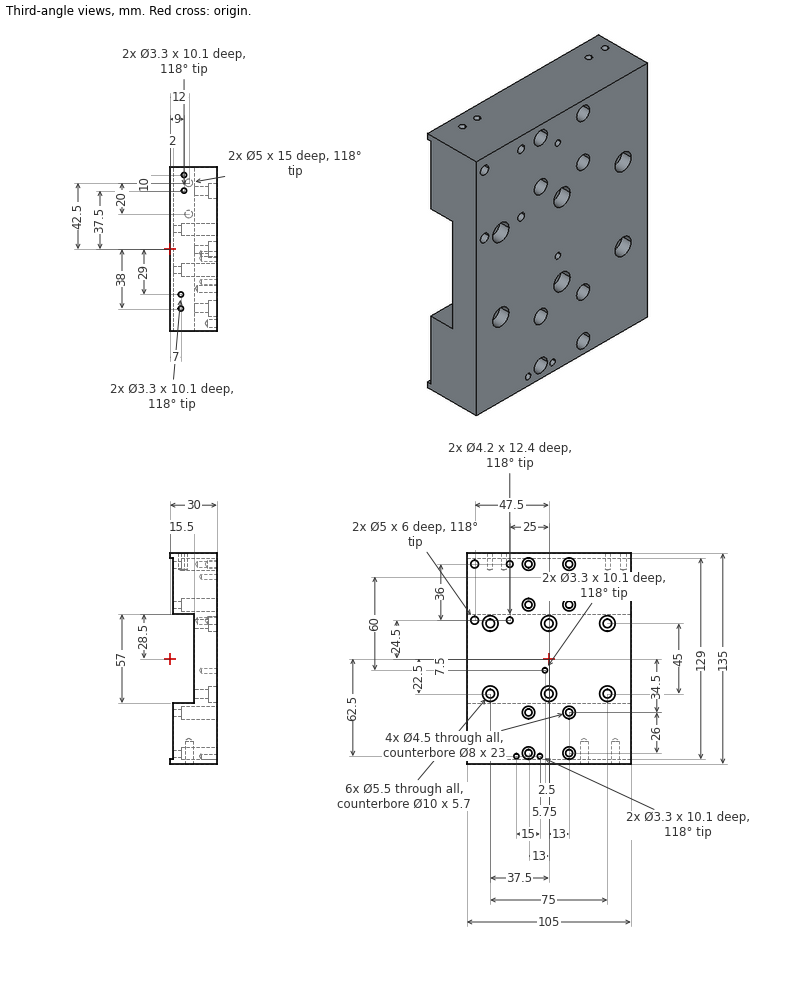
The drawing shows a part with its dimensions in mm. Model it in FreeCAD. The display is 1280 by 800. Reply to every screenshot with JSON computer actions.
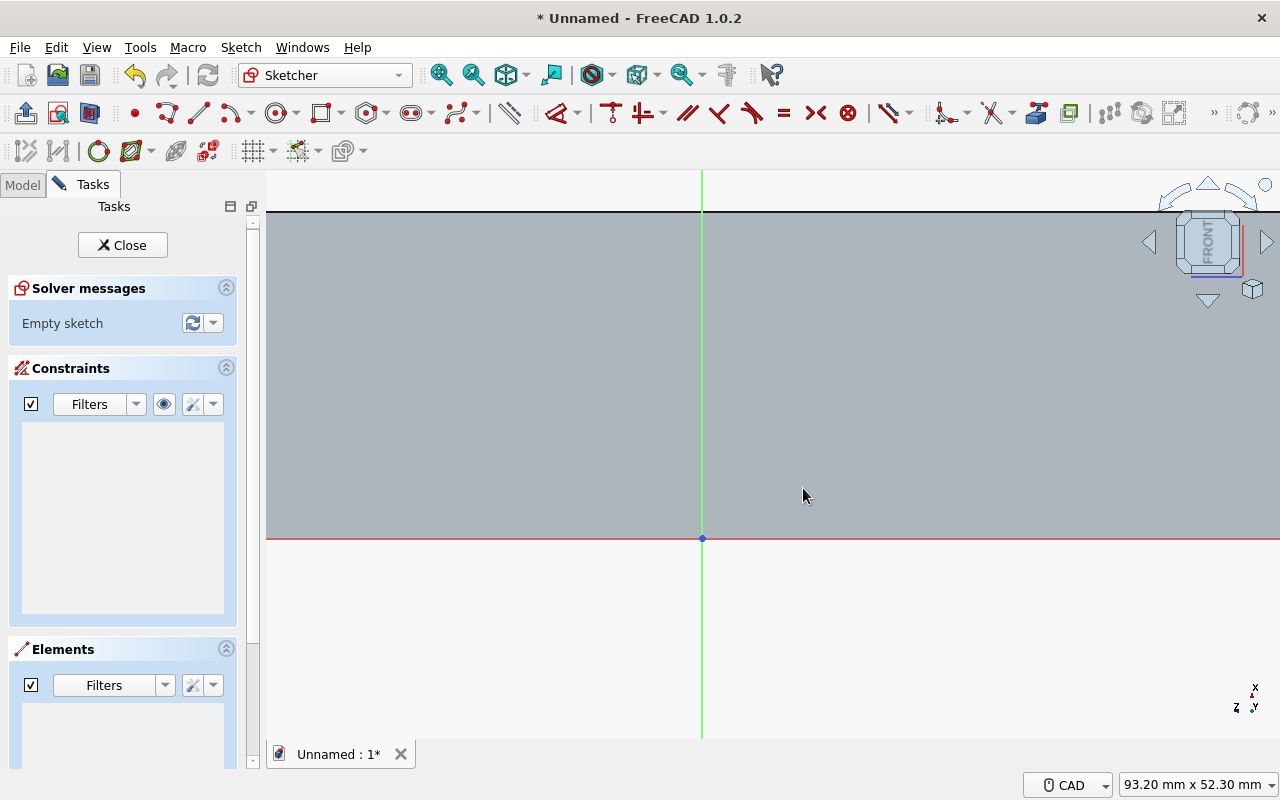
{"action": "left_click", "coordinate": [322, 114]}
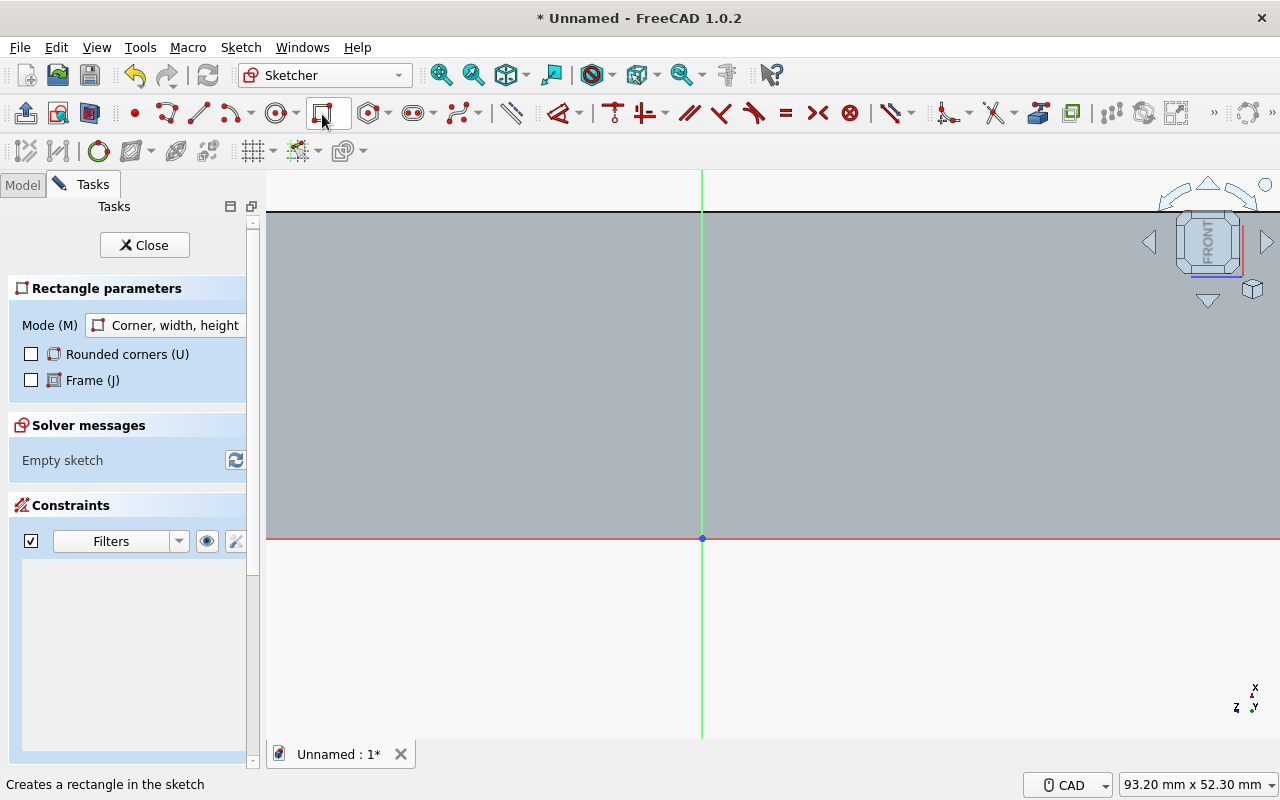
{"action": "left_click", "coordinate": [392, 370]}
{"action": "left_click", "coordinate": [1012, 539]}
{"action": "key", "text": "Escape"}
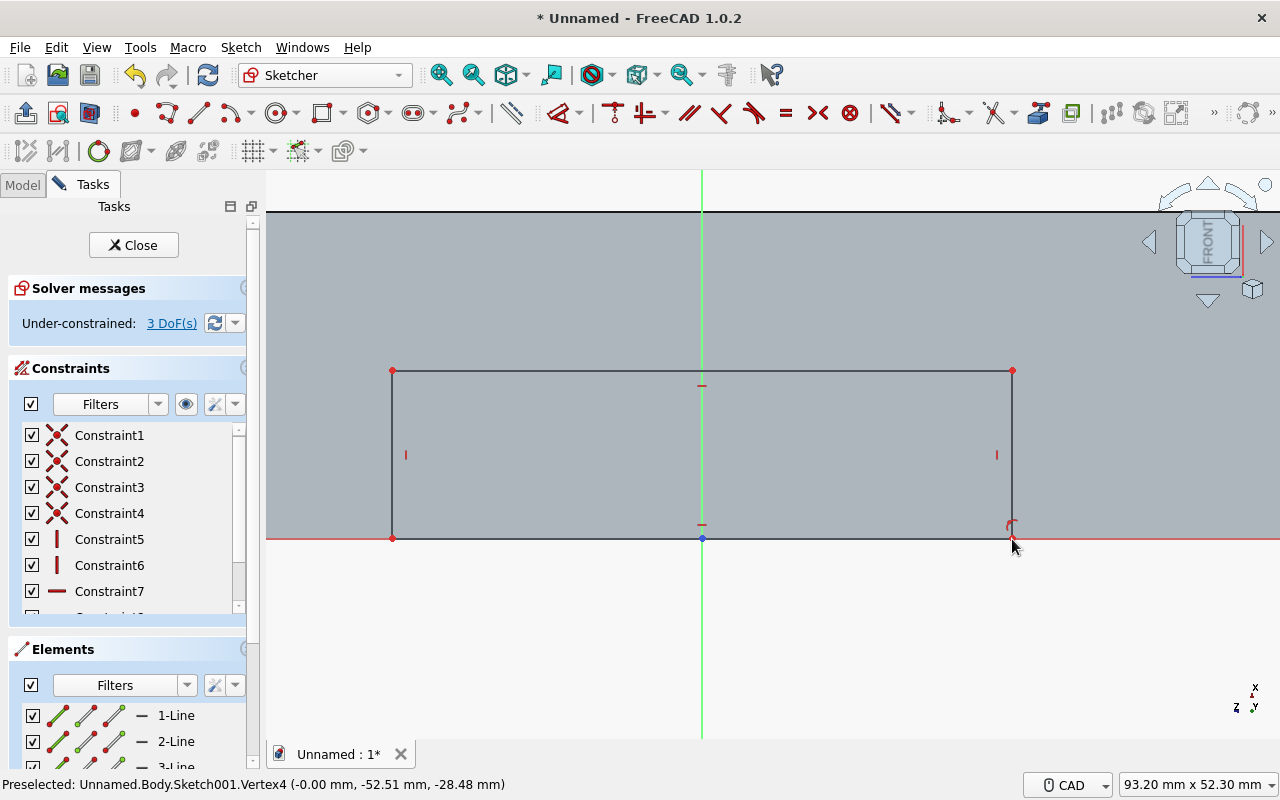
{"action": "left_click", "coordinate": [558, 114]}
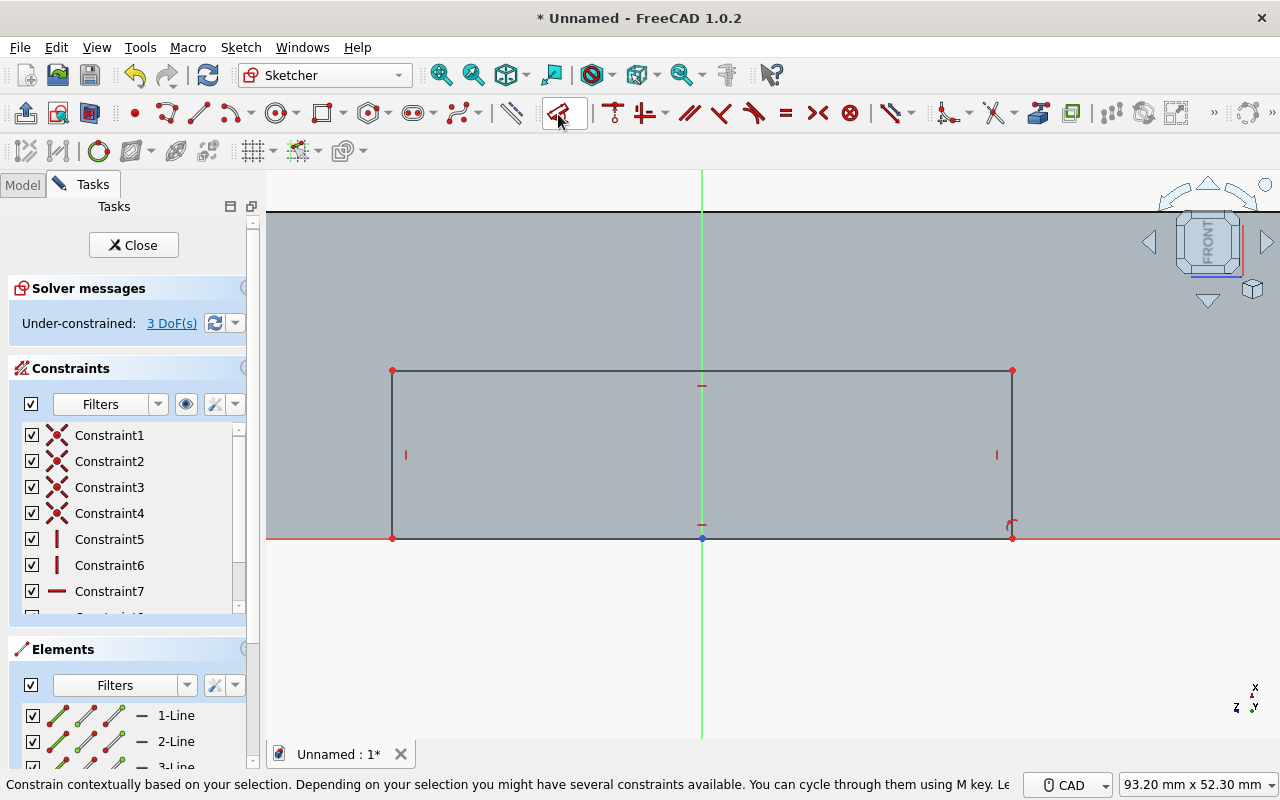
{"action": "left_click", "coordinate": [578, 539]}
{"action": "left_click", "coordinate": [559, 573]}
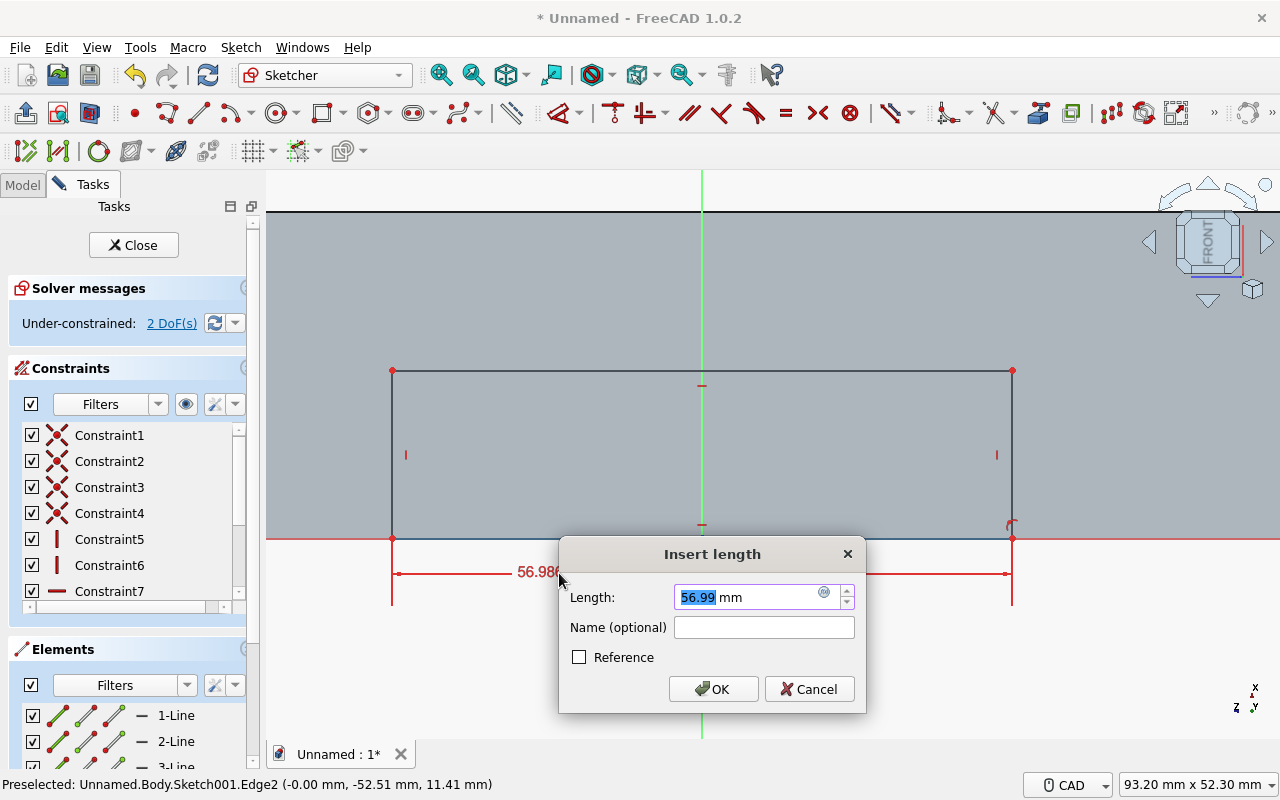
{"action": "type", "text": "57"}
{"action": "key", "text": "Return"}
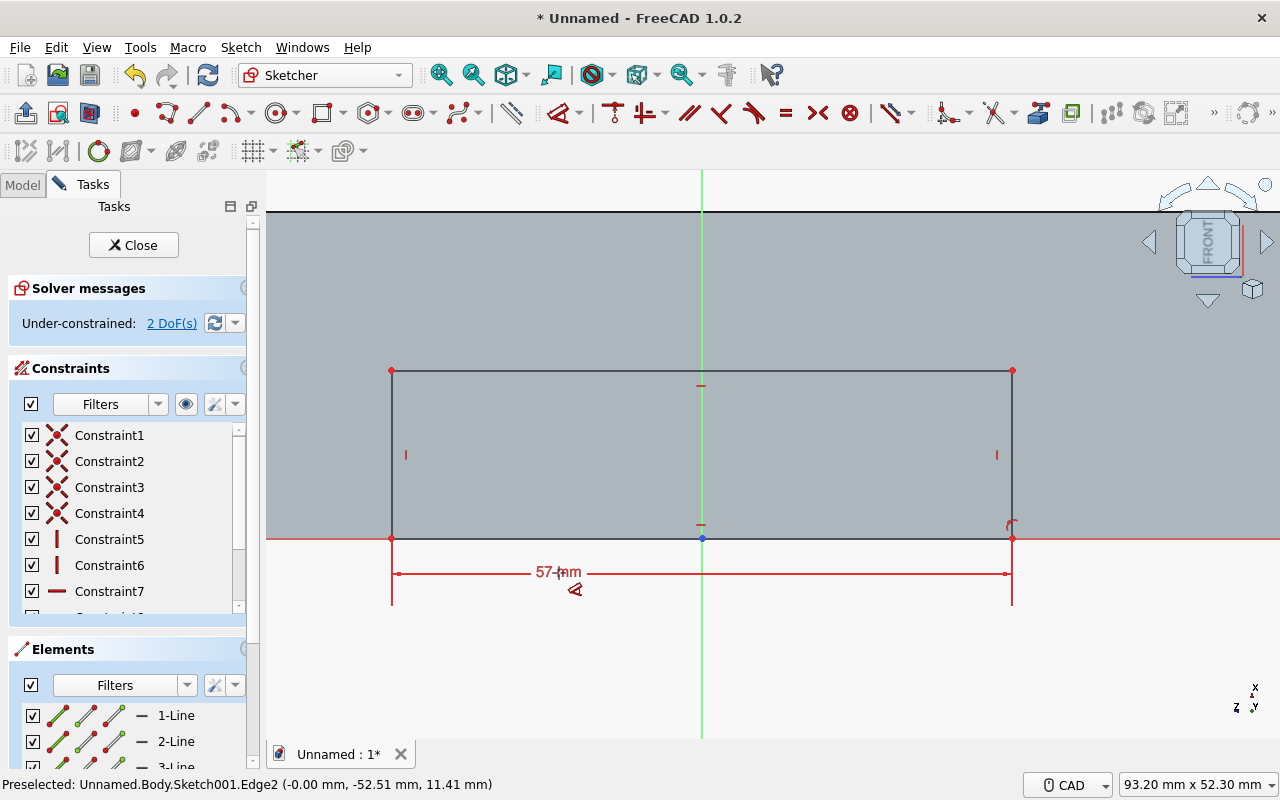
{"action": "left_click", "coordinate": [392, 421]}
{"action": "left_click", "coordinate": [358, 455]}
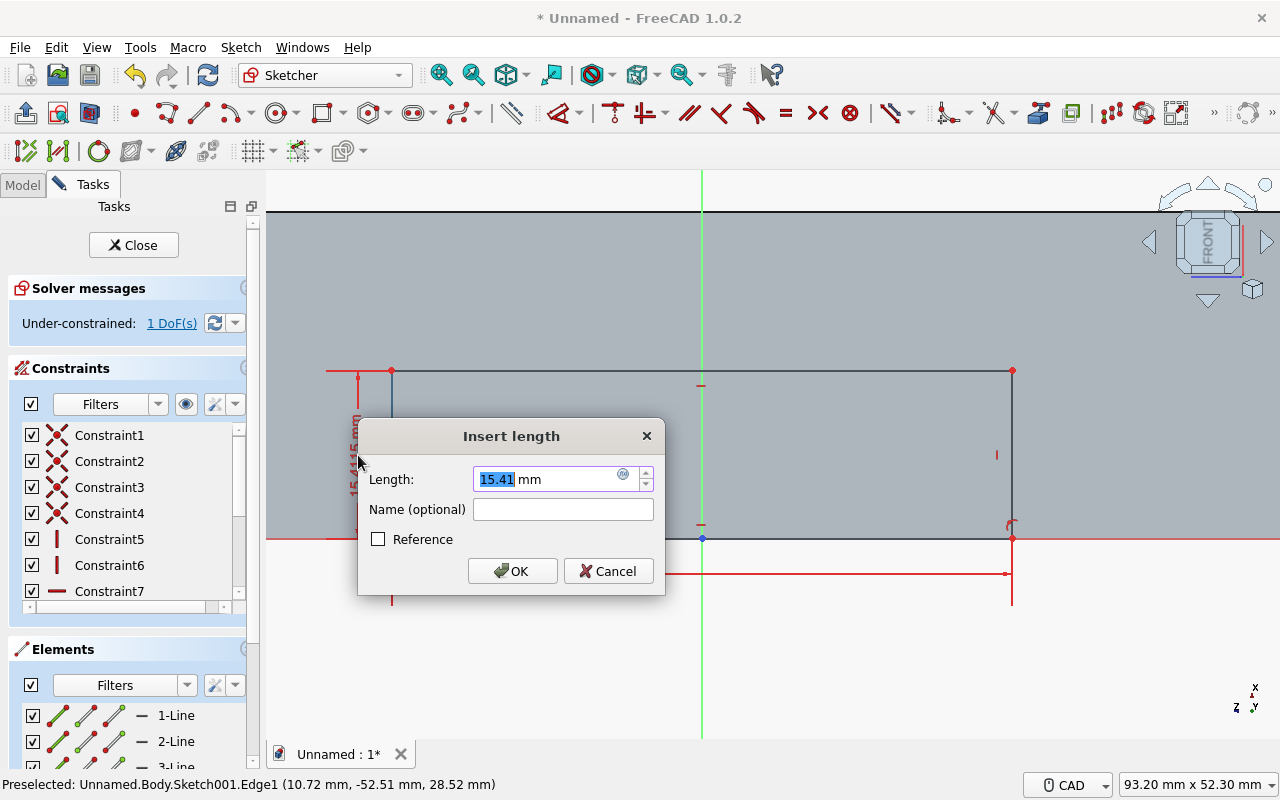
{"action": "type", "text": "15.5"}
{"action": "key", "text": "Return"}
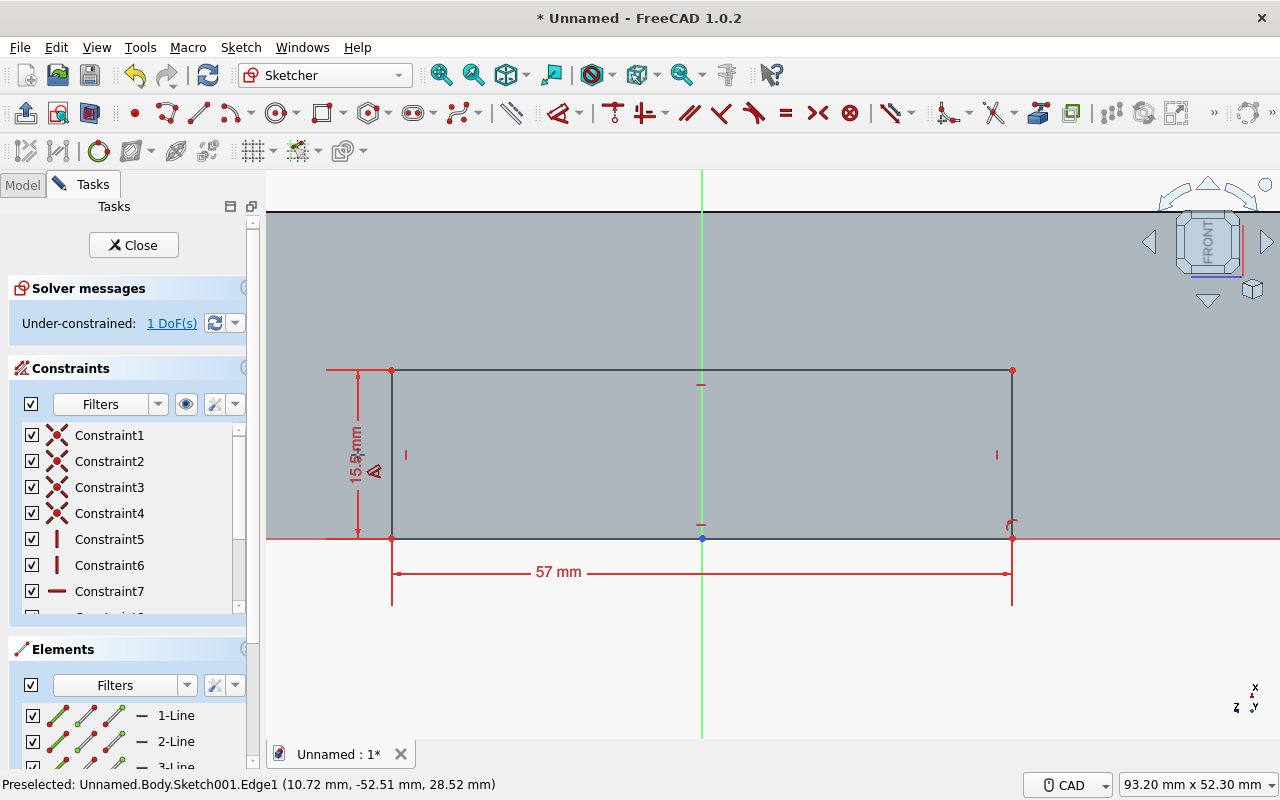
{"action": "left_click", "coordinate": [392, 370]}
{"action": "left_click", "coordinate": [476, 573]}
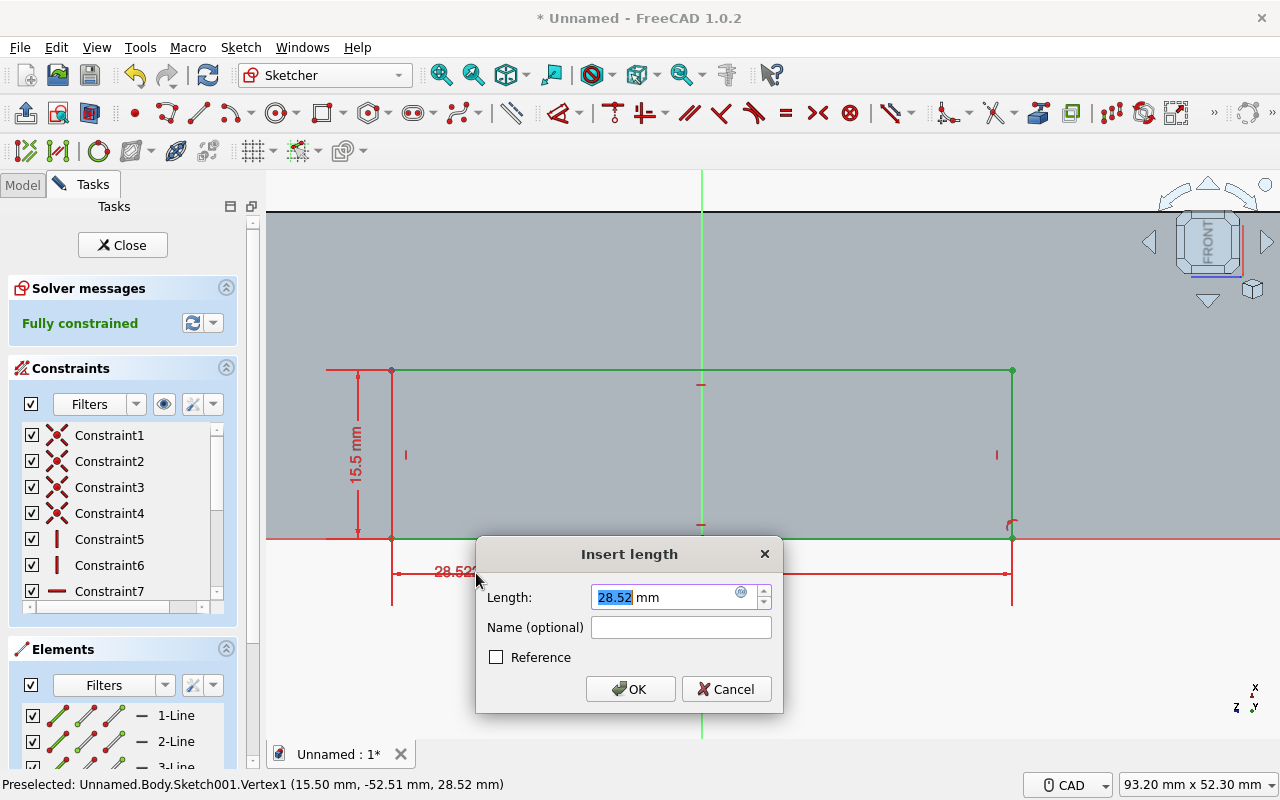
{"action": "type", "text": "28.5"}
{"action": "key", "text": "Return"}
{"action": "key", "text": "Escape"}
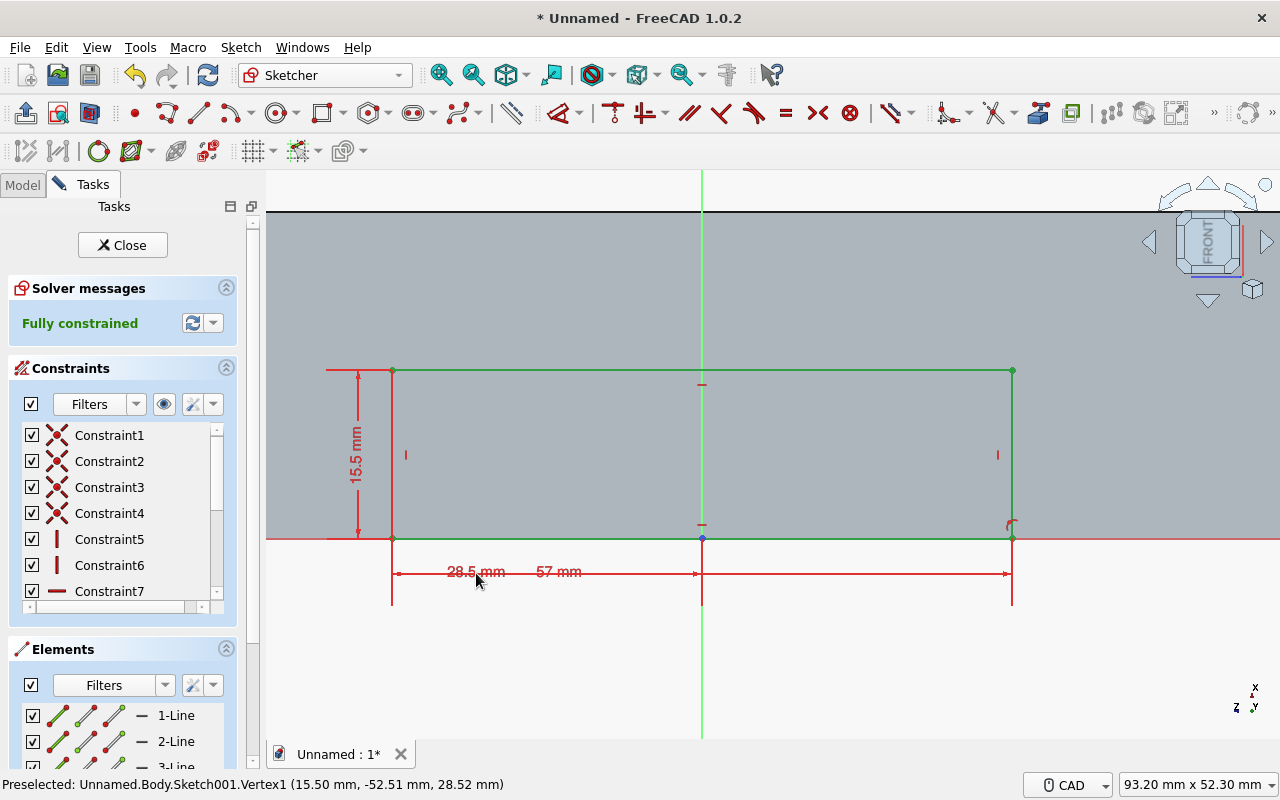
{"action": "left_click", "coordinate": [123, 245]}